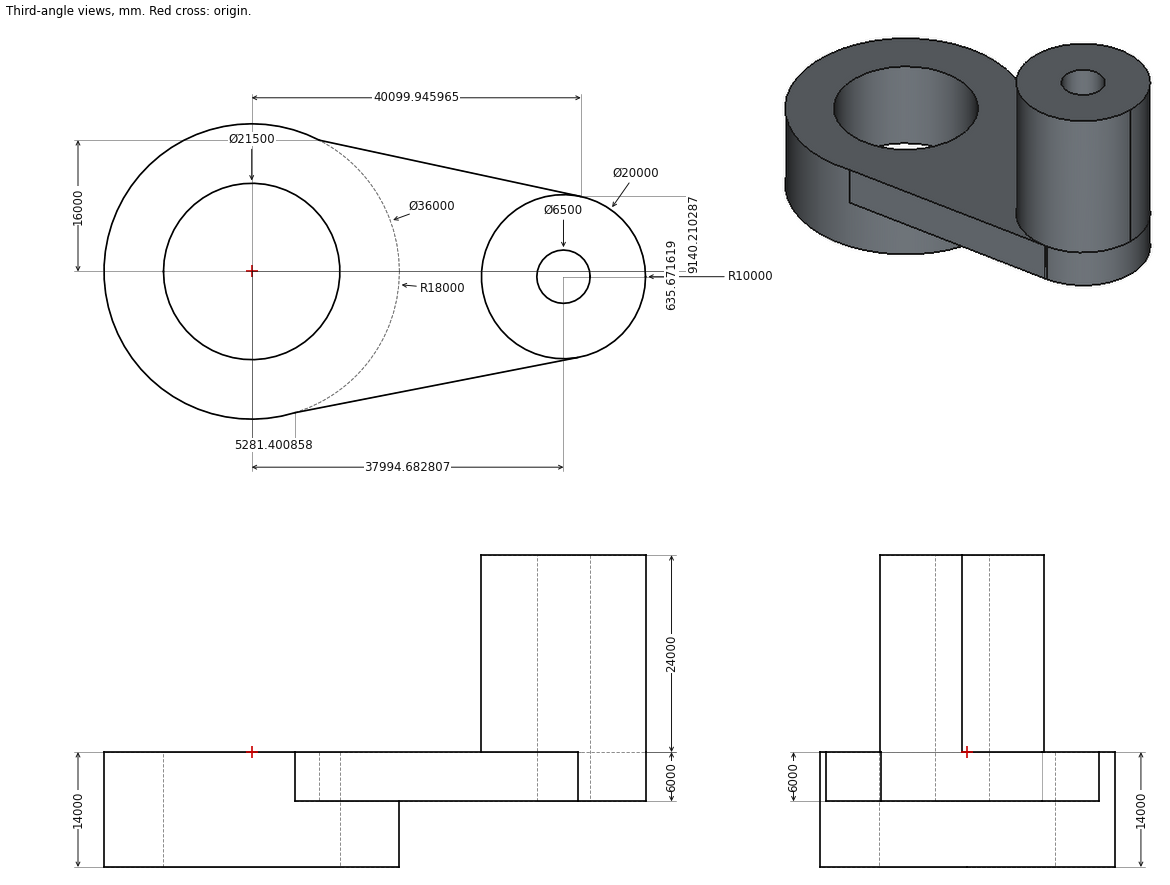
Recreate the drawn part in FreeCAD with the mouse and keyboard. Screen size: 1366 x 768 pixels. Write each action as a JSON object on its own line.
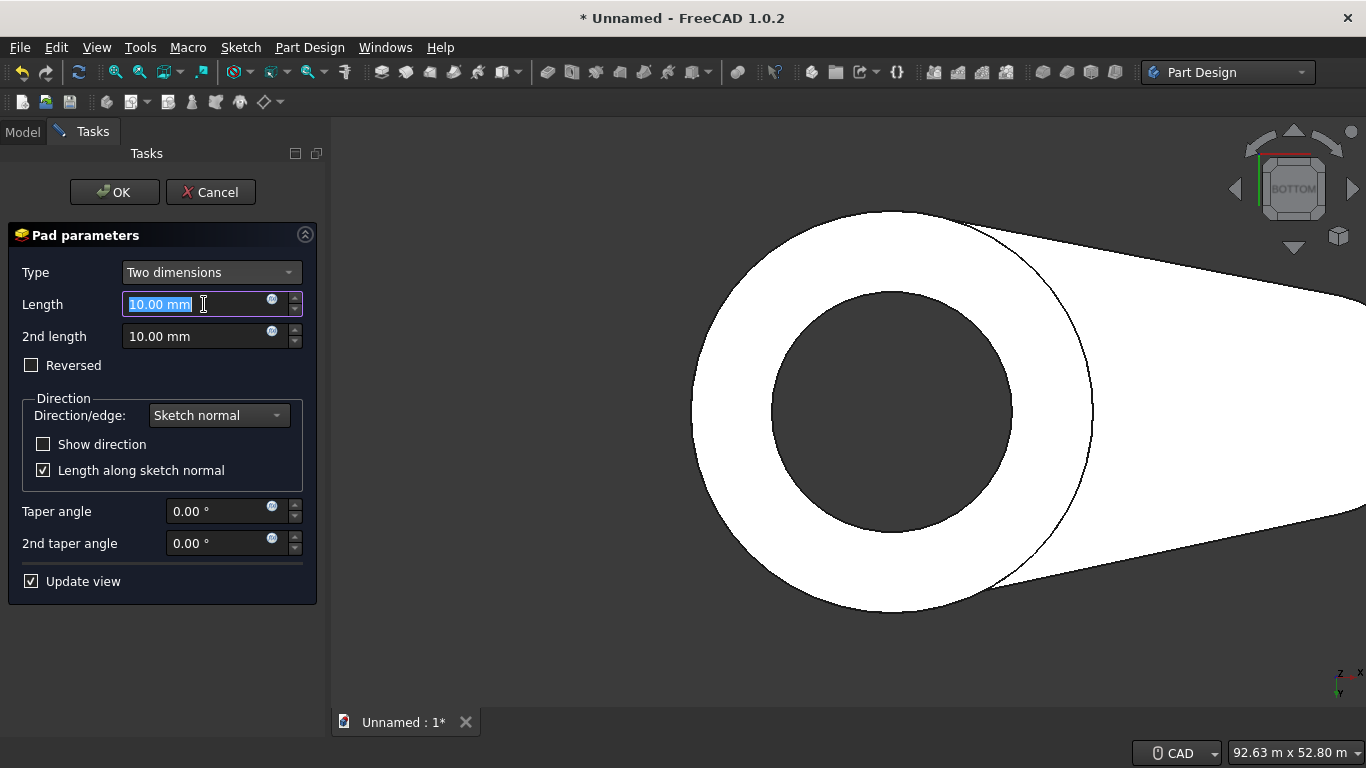
{"action": "type", "text": "24000"}
{"action": "key", "text": "Tab"}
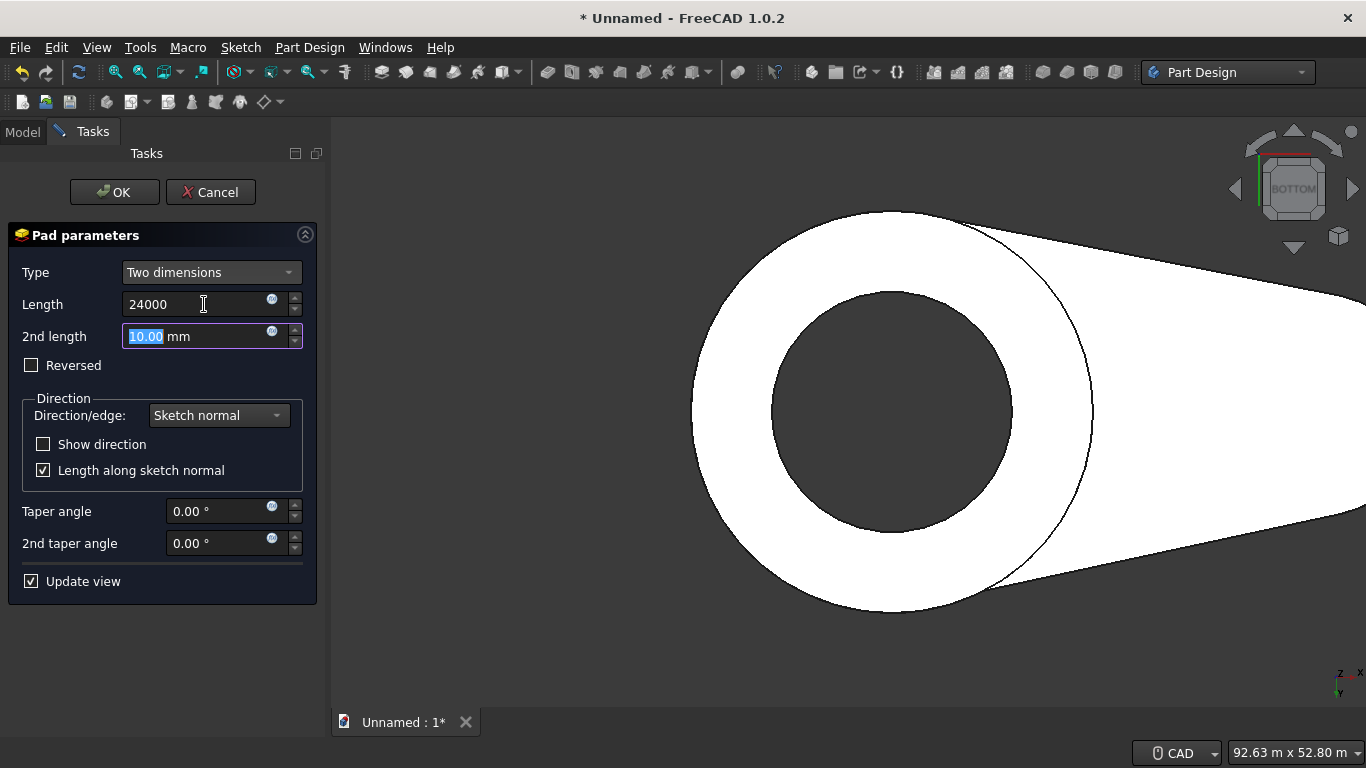
{"action": "type", "text": "6000"}
{"action": "key", "text": "Tab"}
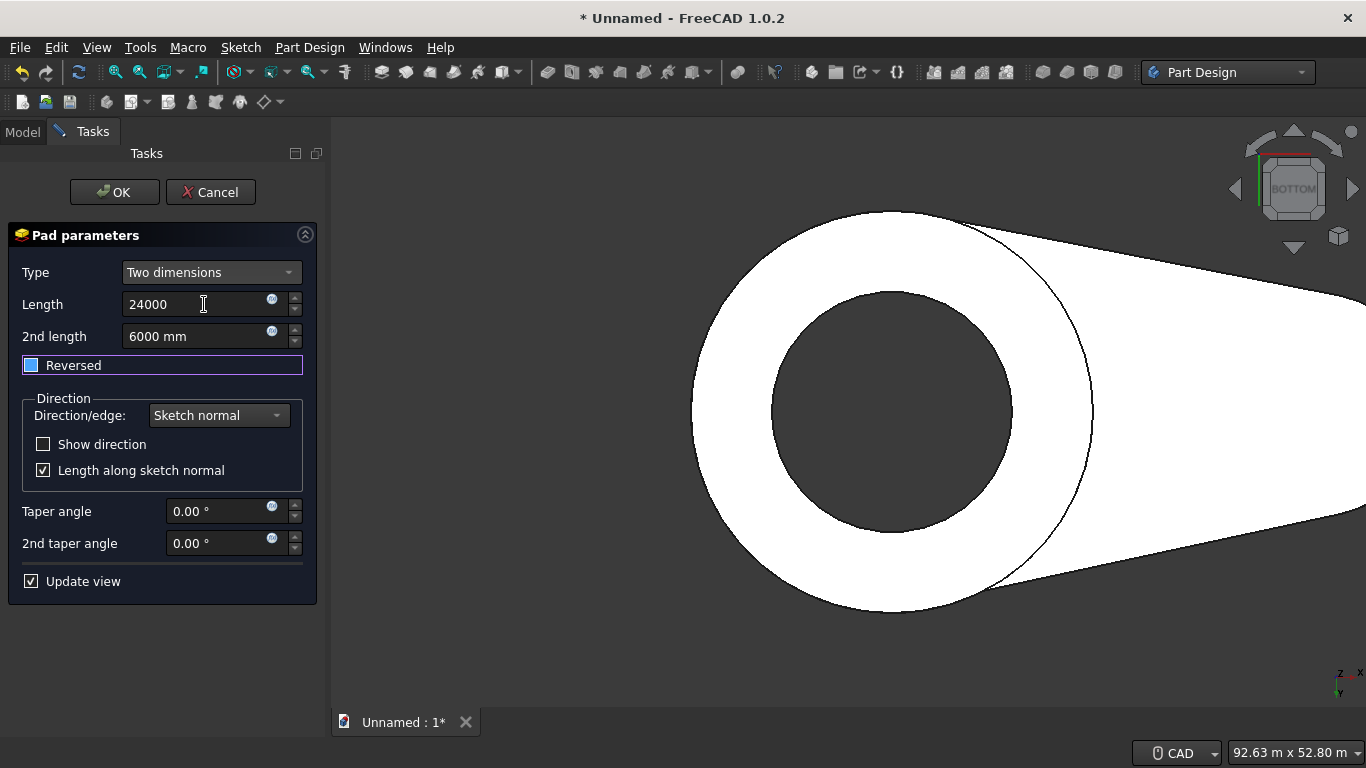
{"action": "left_click", "coordinate": [115, 192]}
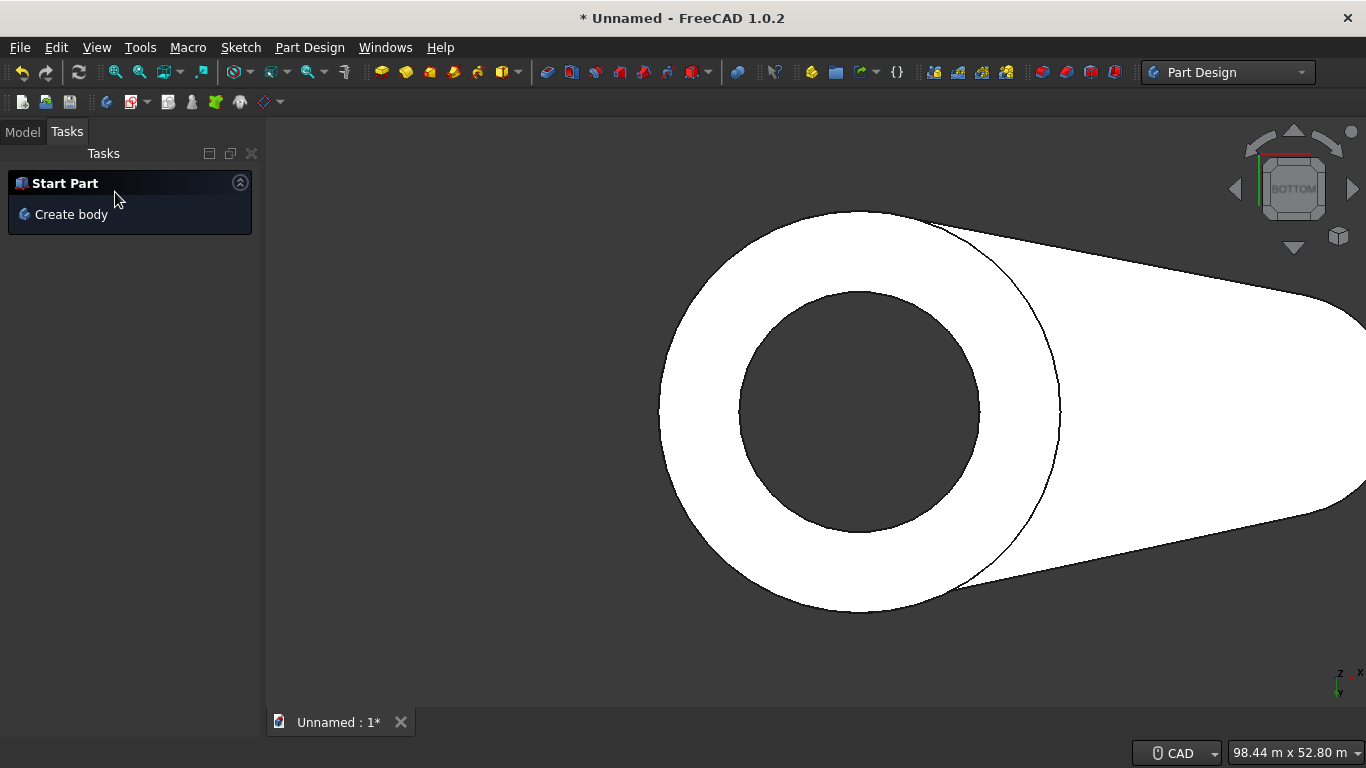
{"action": "left_click", "coordinate": [116, 72]}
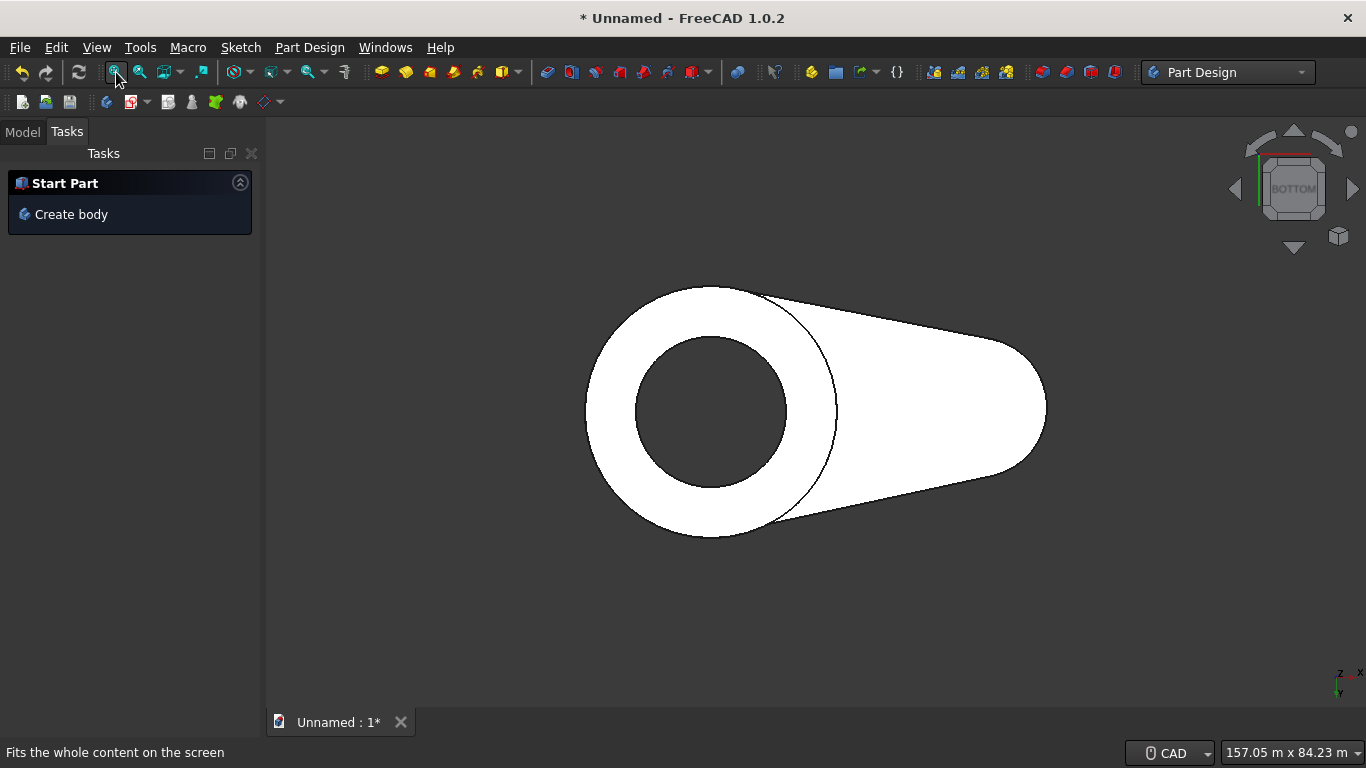
{"action": "key", "text": "0"}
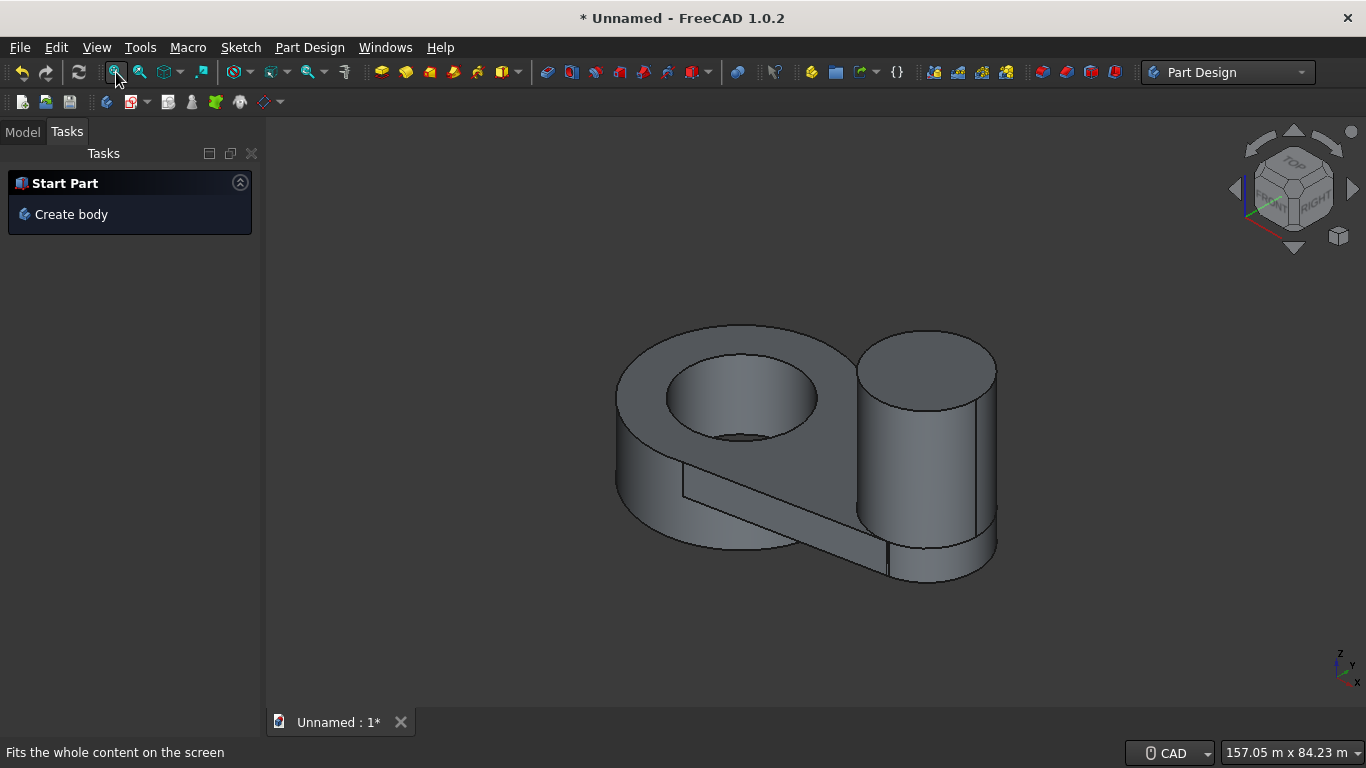
{"action": "left_click", "coordinate": [927, 370]}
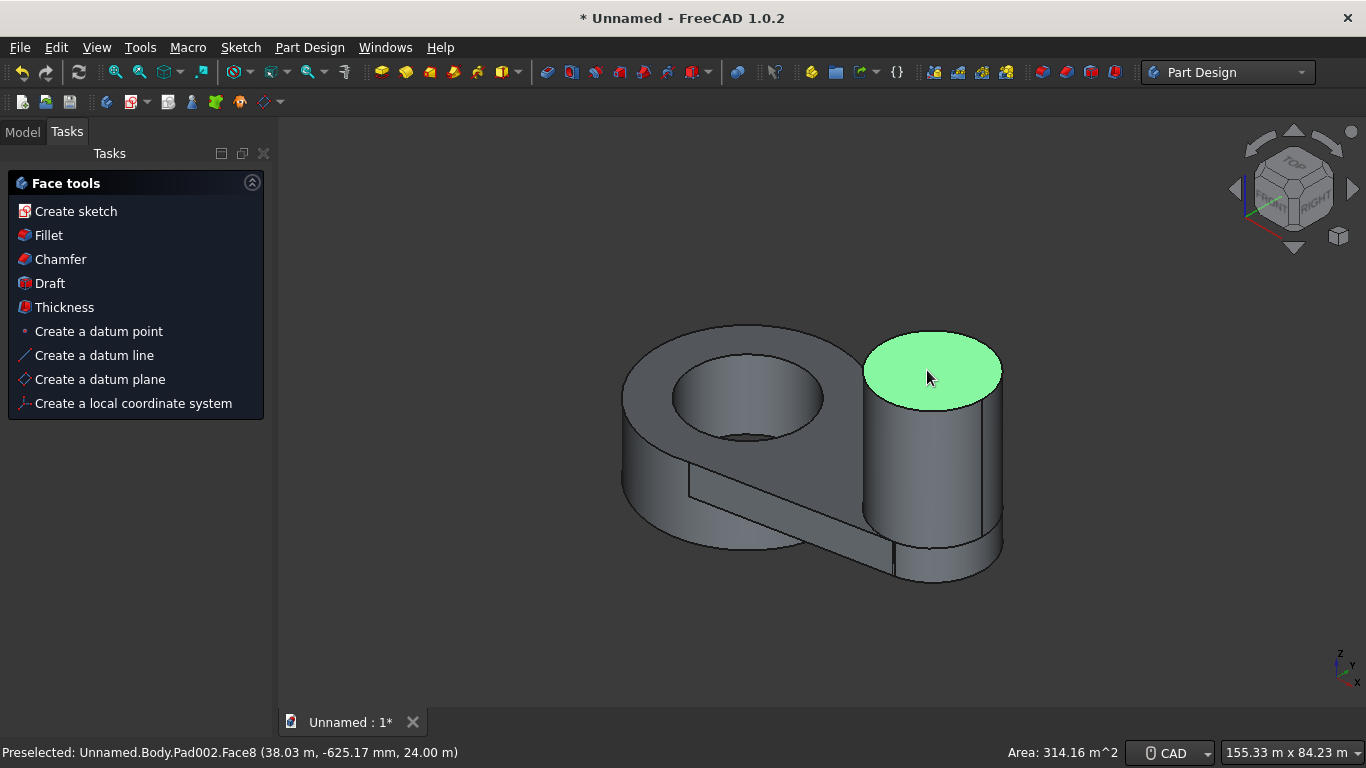
{"action": "left_click", "coordinate": [132, 102]}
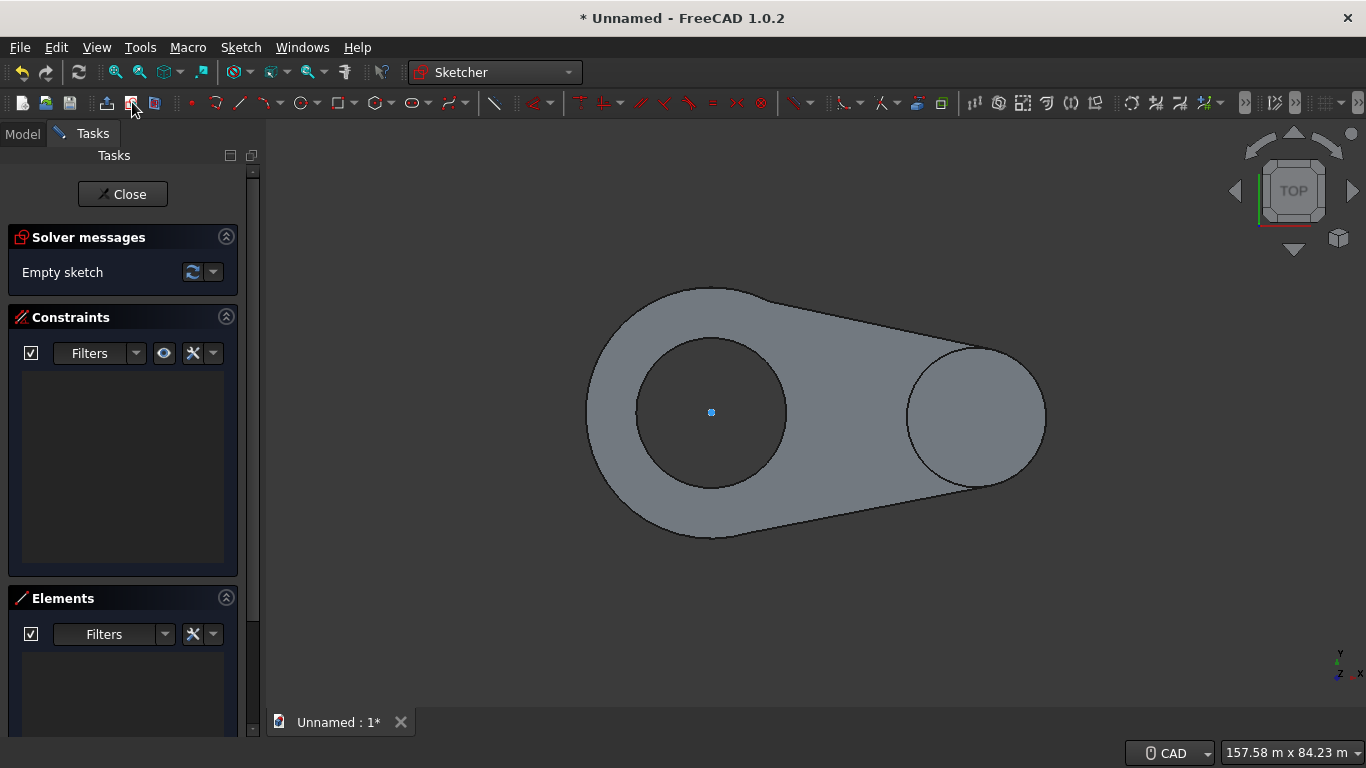
{"action": "scroll", "coordinate": [1005, 418], "scroll_direction": "up", "scroll_amount": 11}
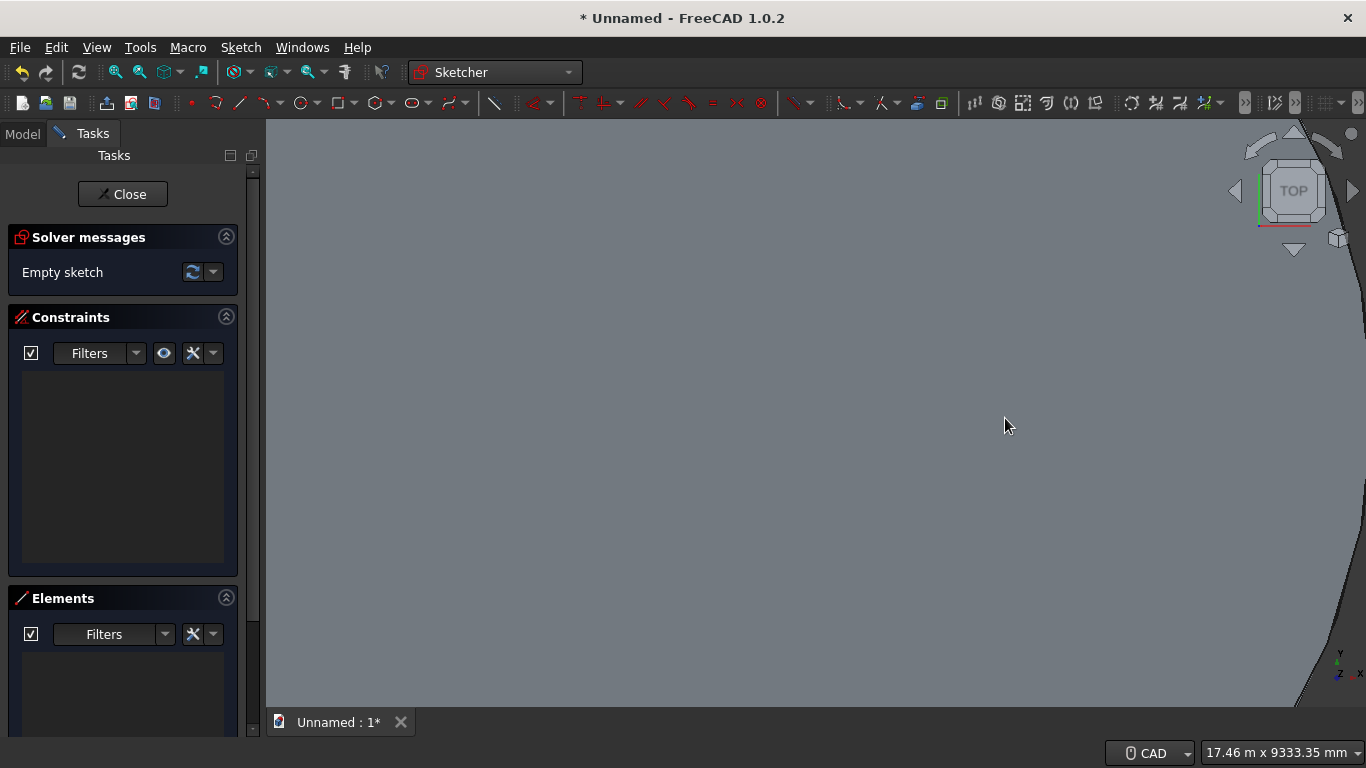
{"action": "left_click", "coordinate": [302, 104]}